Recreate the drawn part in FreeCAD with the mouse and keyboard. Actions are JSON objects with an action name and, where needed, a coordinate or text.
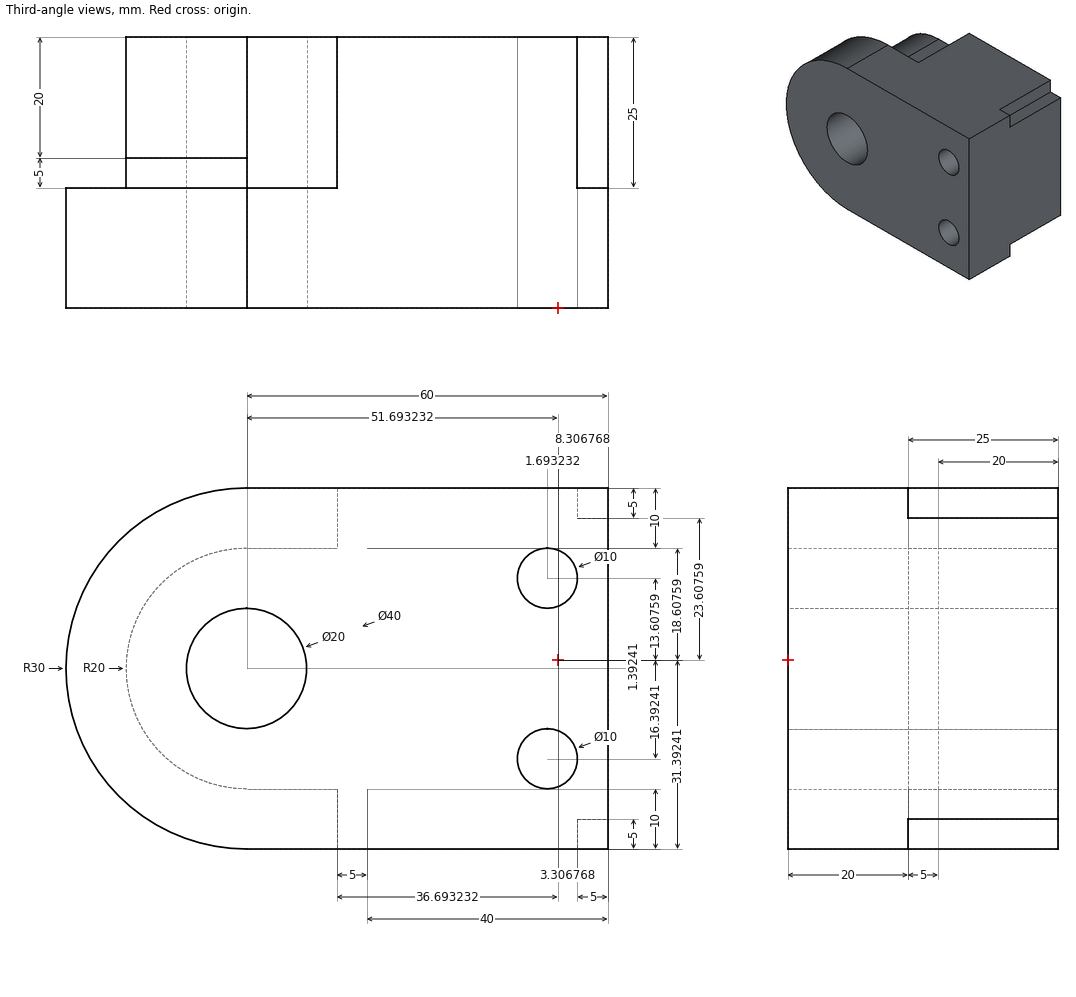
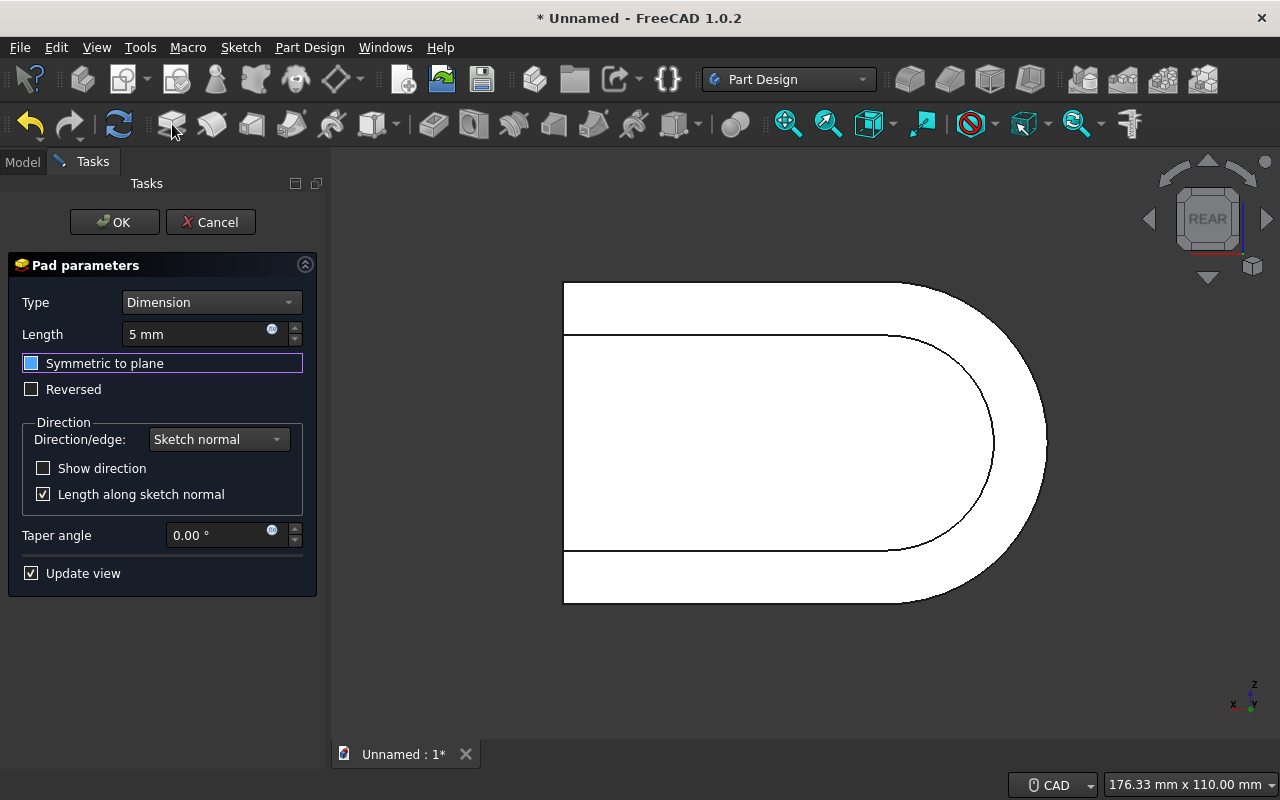
{"action": "left_click", "coordinate": [115, 222]}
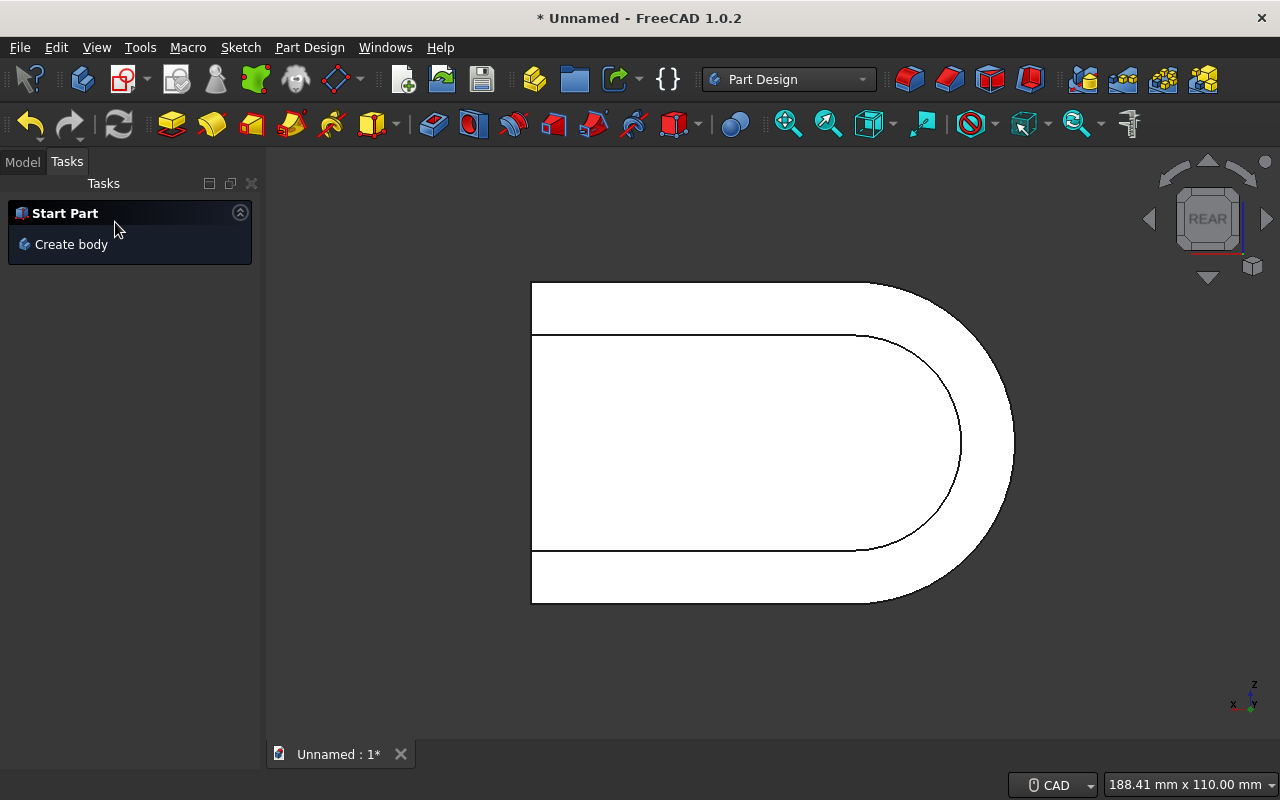
{"action": "left_click", "coordinate": [685, 442]}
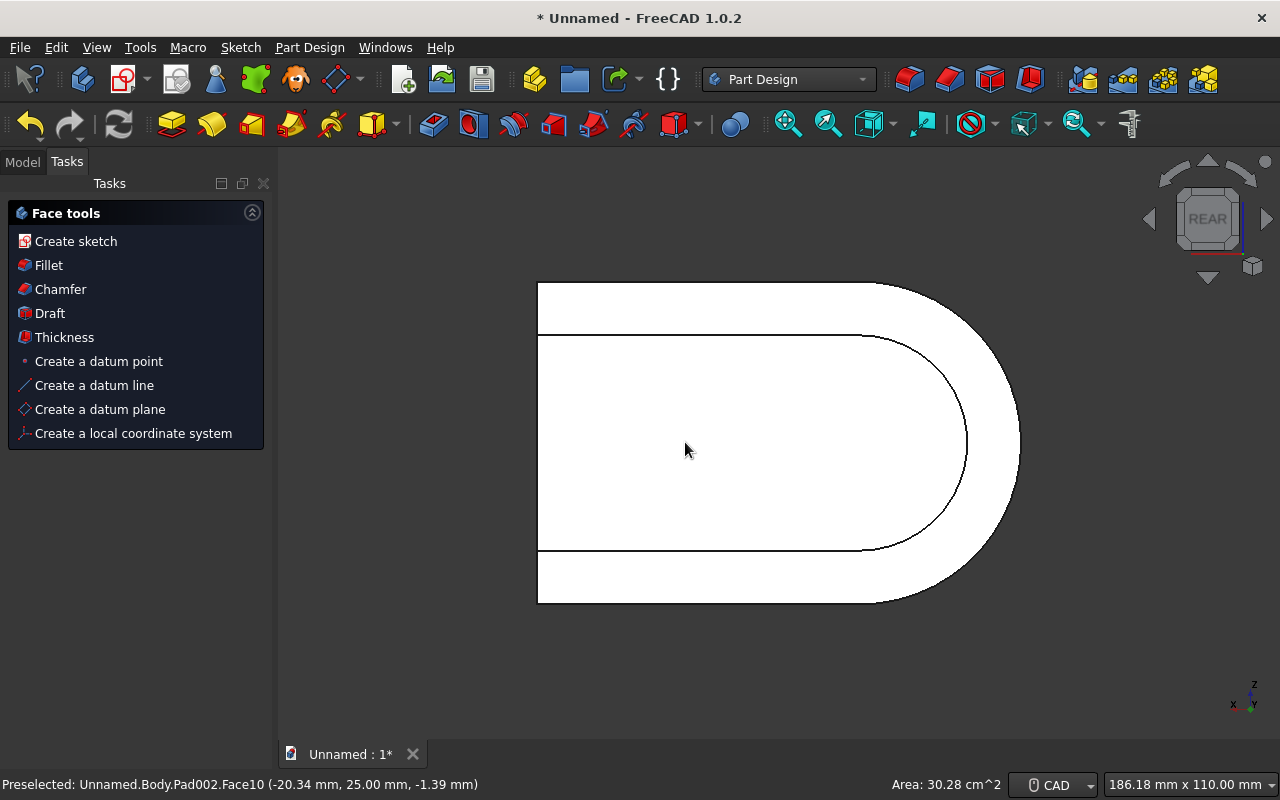
{"action": "left_click", "coordinate": [124, 80]}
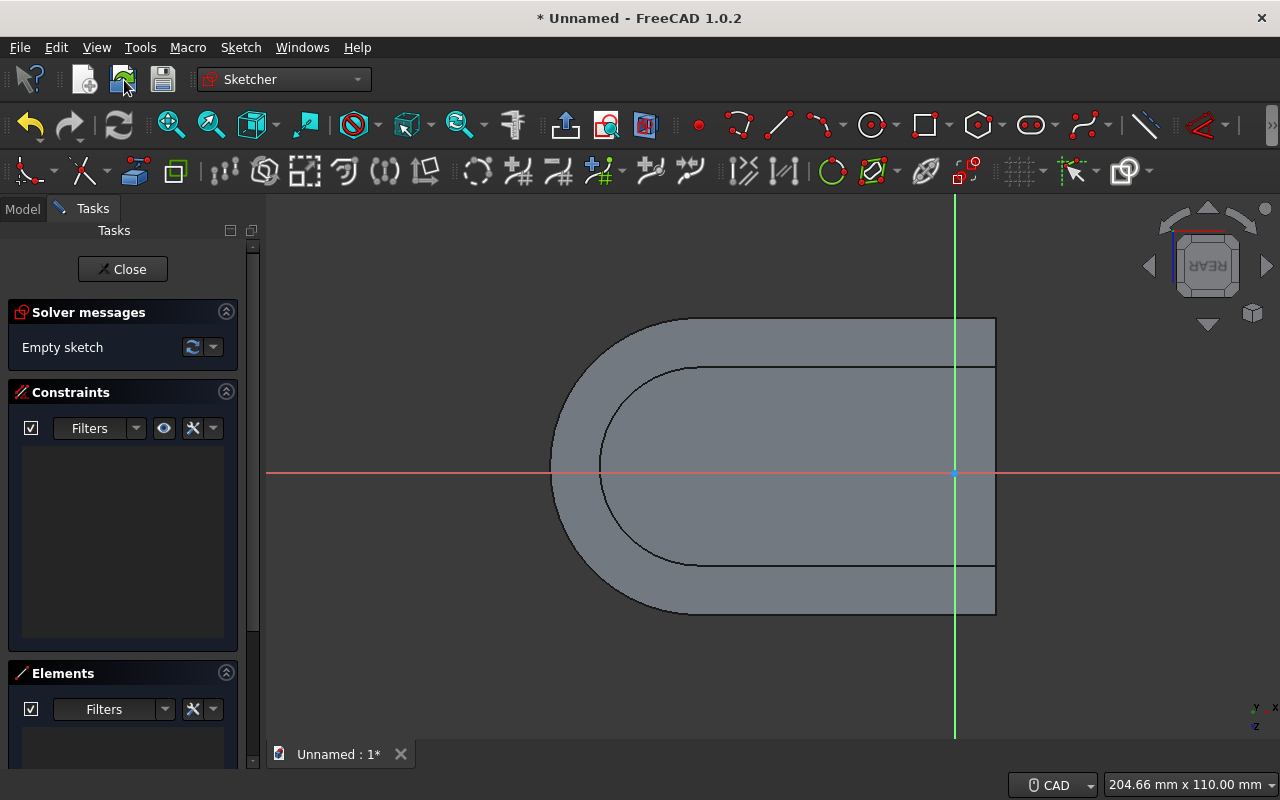
{"action": "scroll", "coordinate": [925, 466], "scroll_direction": "up", "scroll_amount": 2}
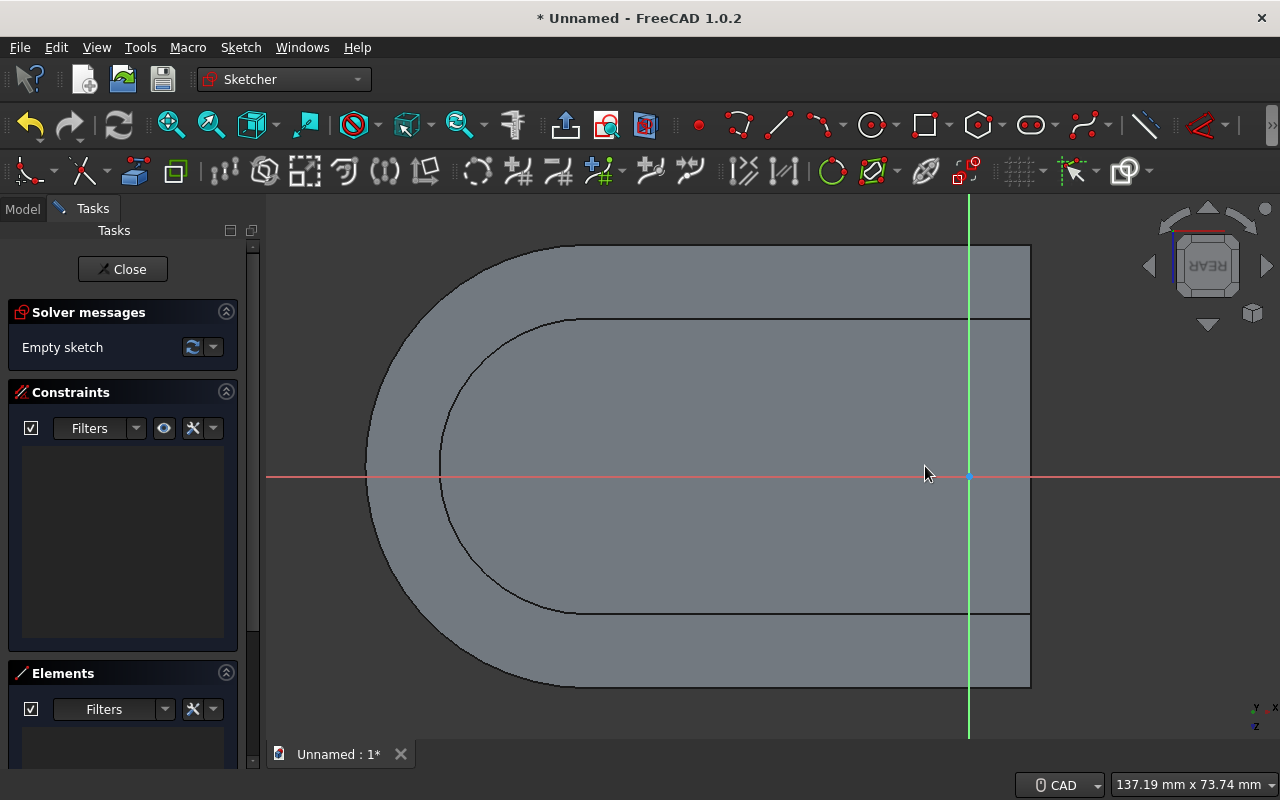
{"action": "key", "text": "g c"}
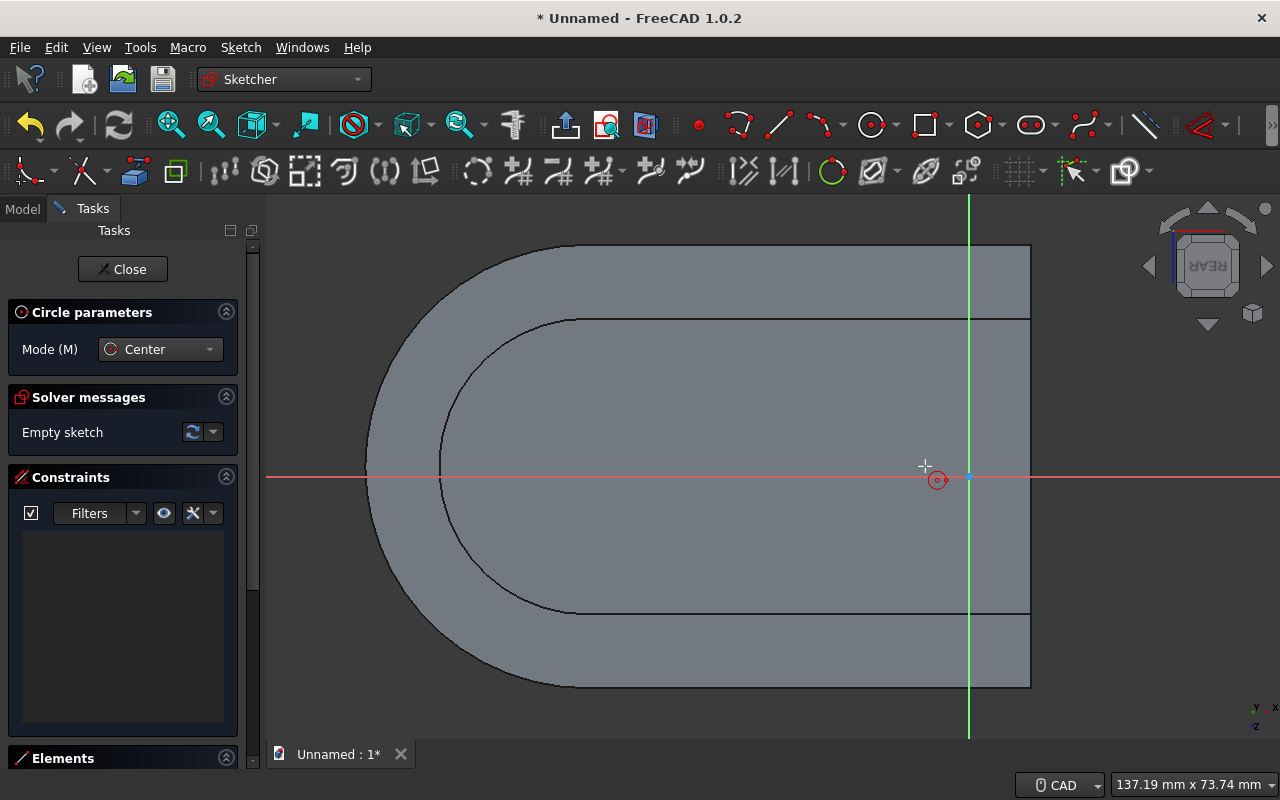
{"action": "scroll", "coordinate": [587, 466], "scroll_direction": "up", "scroll_amount": 3}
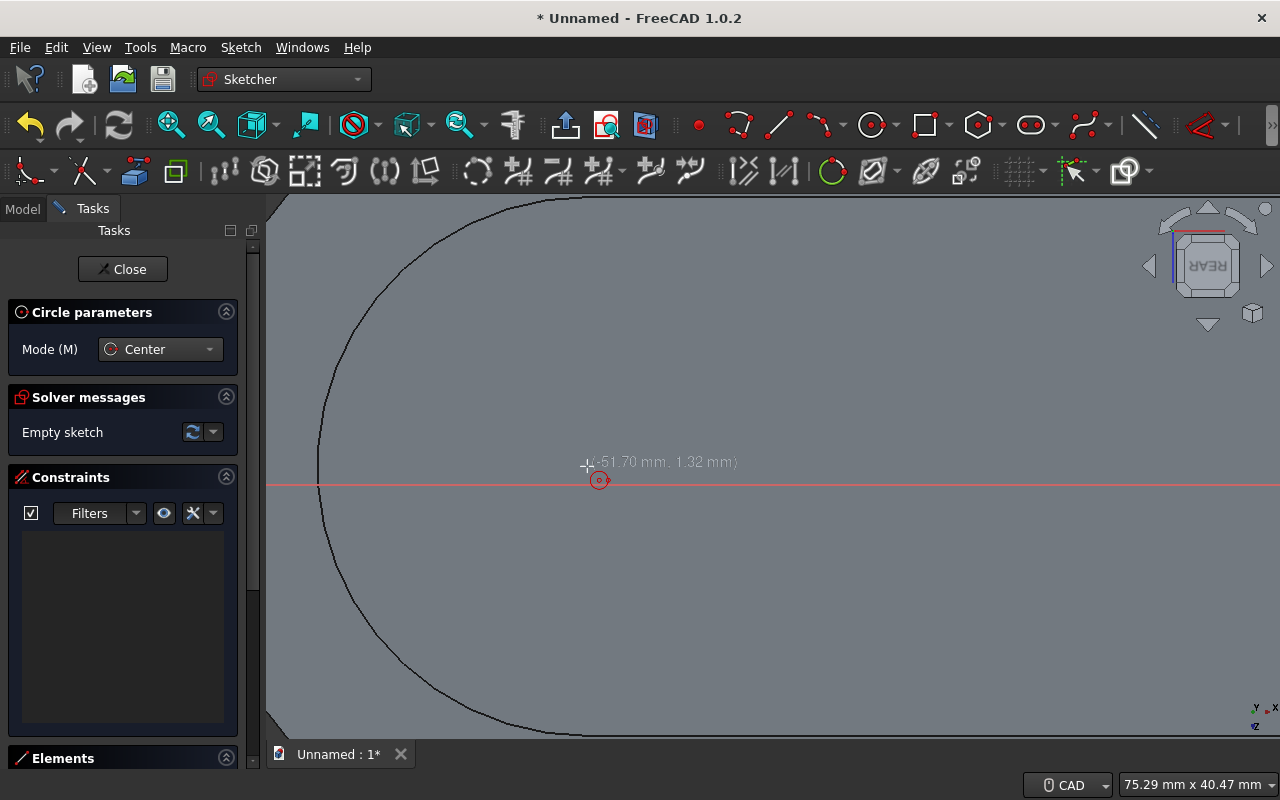
{"action": "left_click", "coordinate": [587, 466]}
{"action": "left_click", "coordinate": [777, 276]}
{"action": "key", "text": "Escape"}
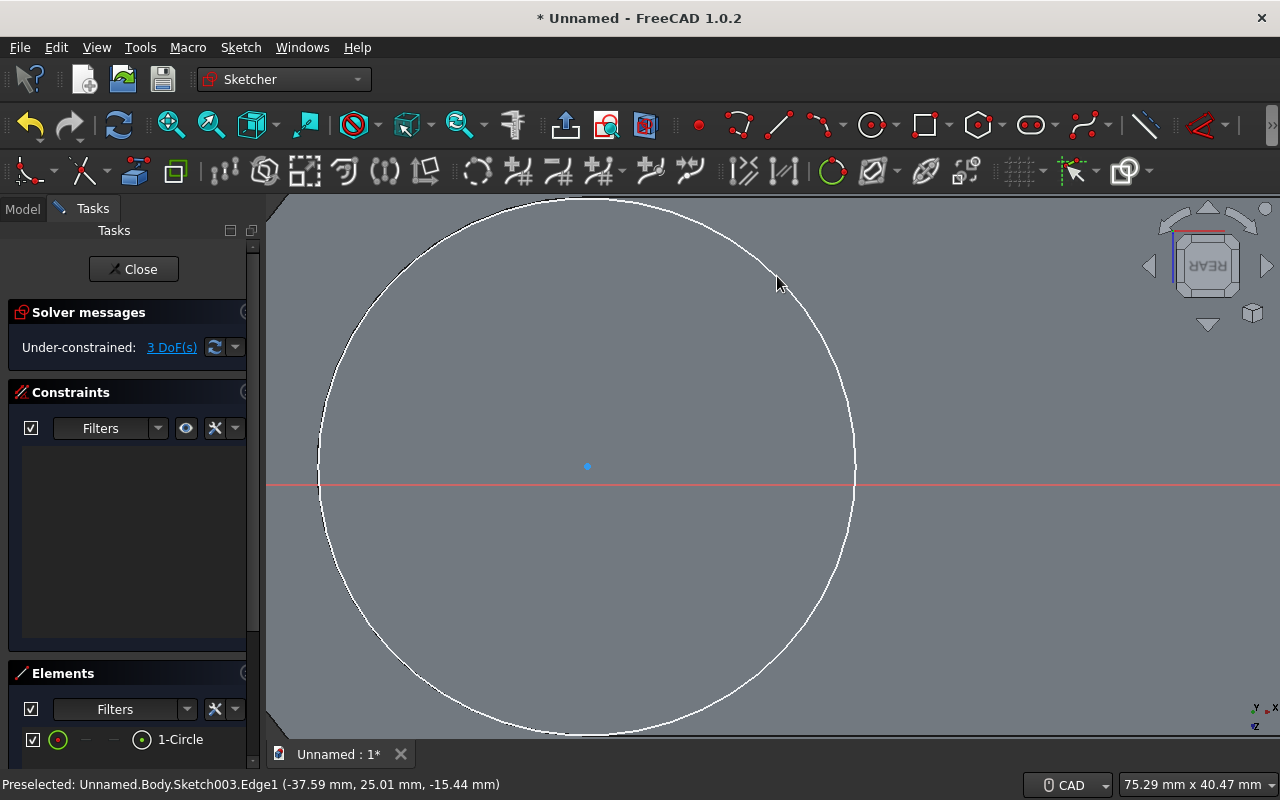
{"action": "key", "text": "d"}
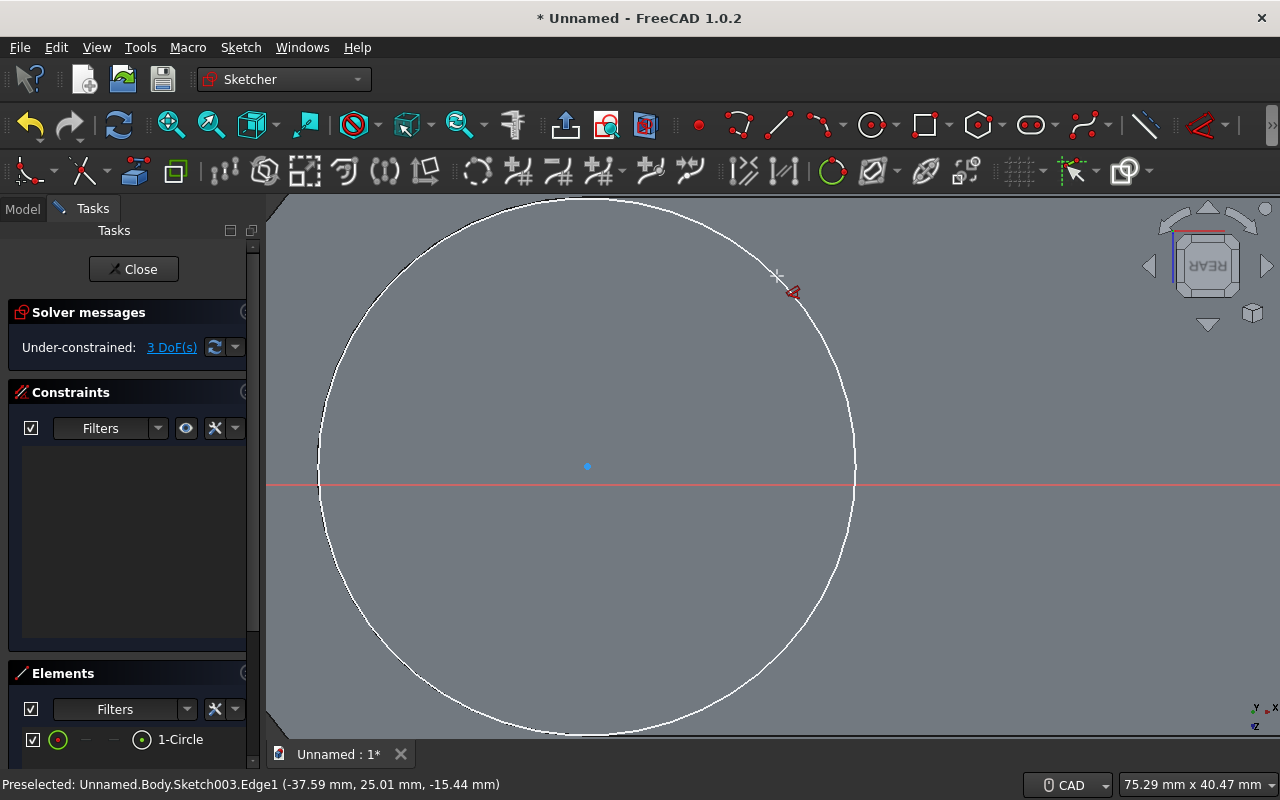
{"action": "left_click", "coordinate": [776, 276]}
{"action": "left_click", "coordinate": [799, 253]}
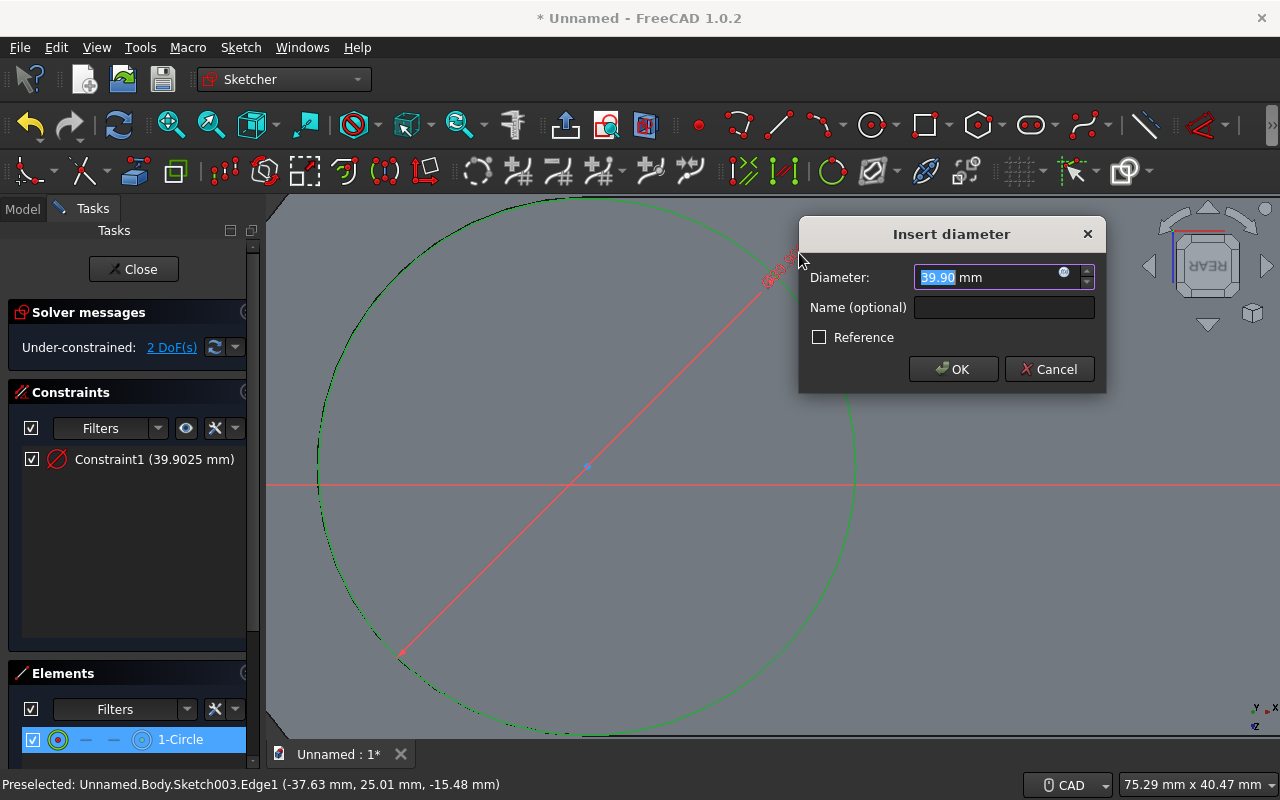
{"action": "type", "text": "40"}
{"action": "key", "text": "Return"}